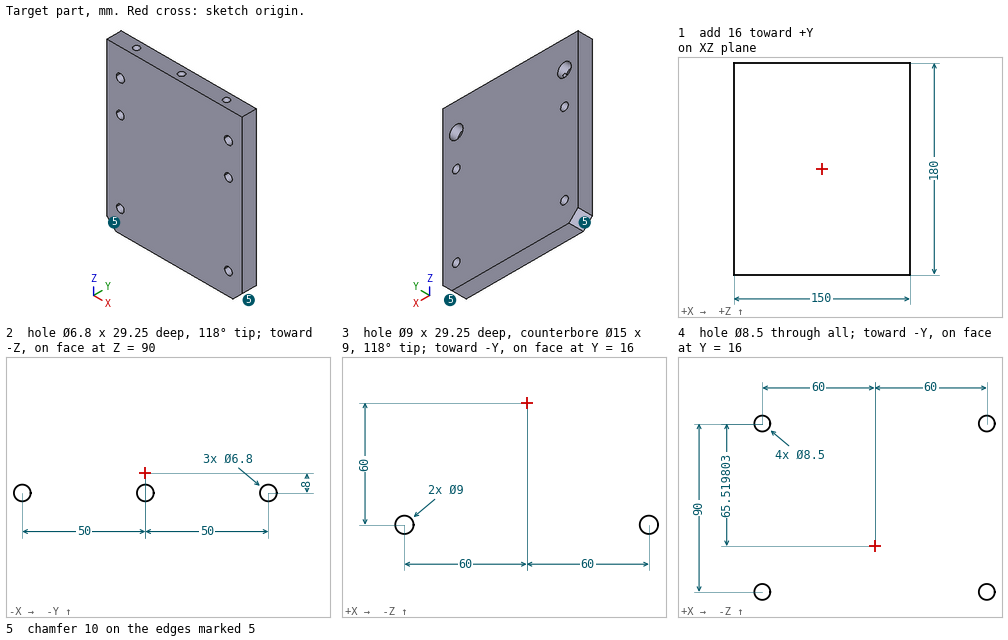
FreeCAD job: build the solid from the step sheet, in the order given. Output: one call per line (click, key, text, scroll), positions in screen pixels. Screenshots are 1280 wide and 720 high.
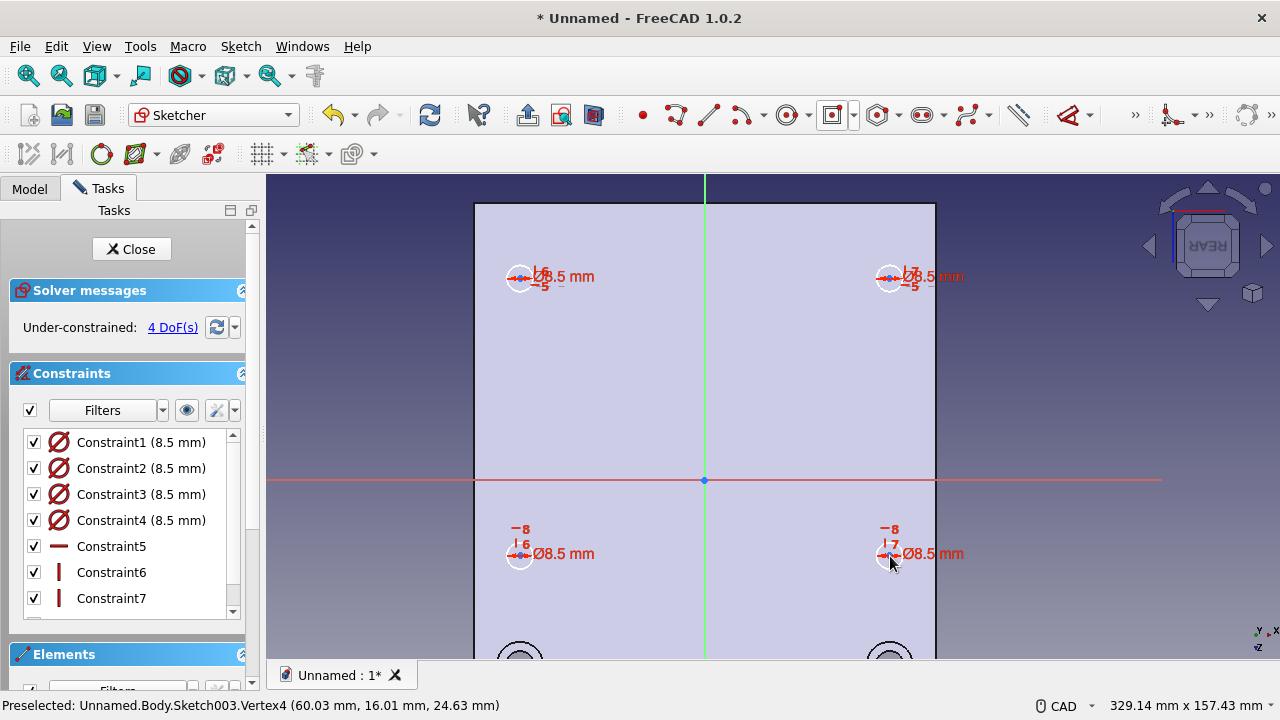
click(1068, 116)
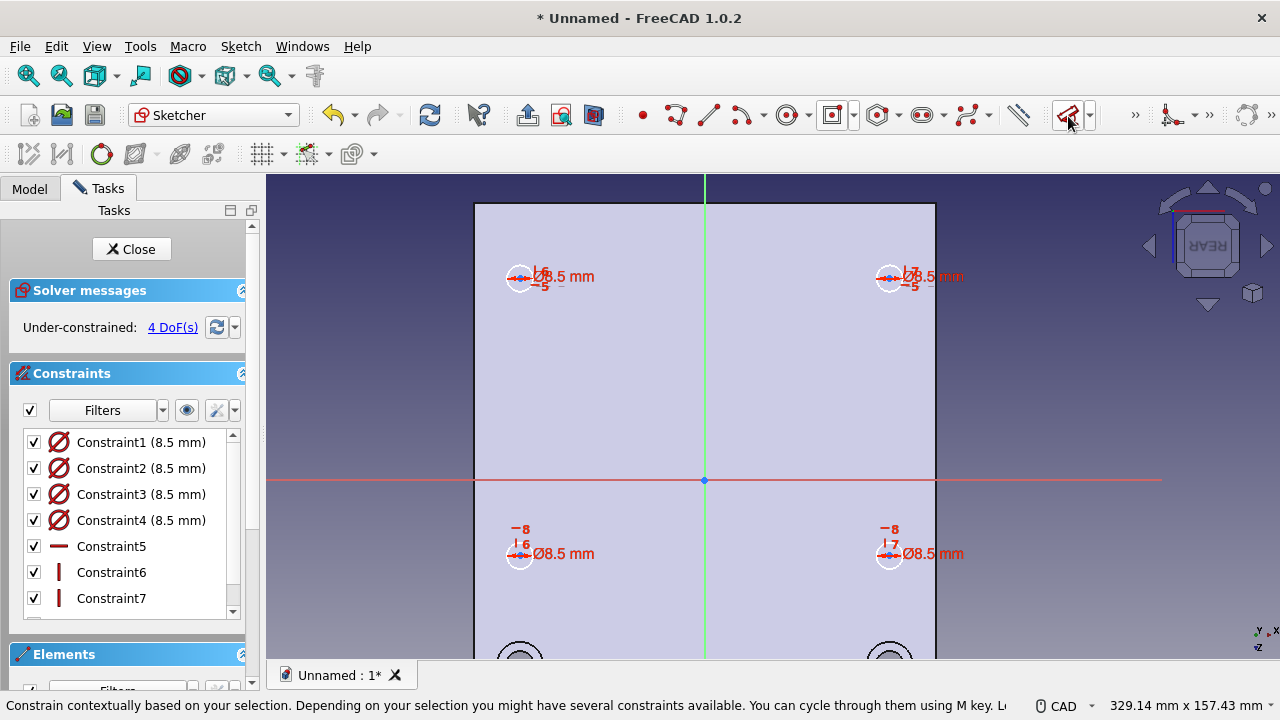
click(520, 279)
click(612, 245)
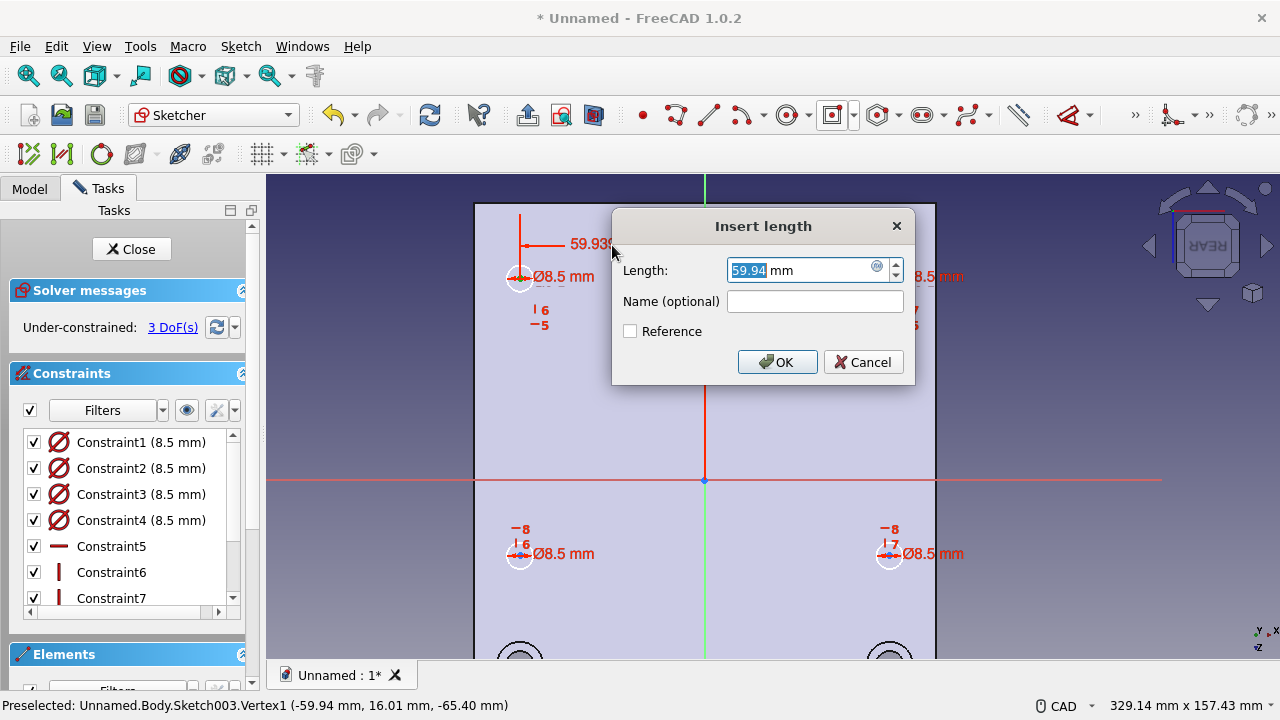
text(60)
key(Return)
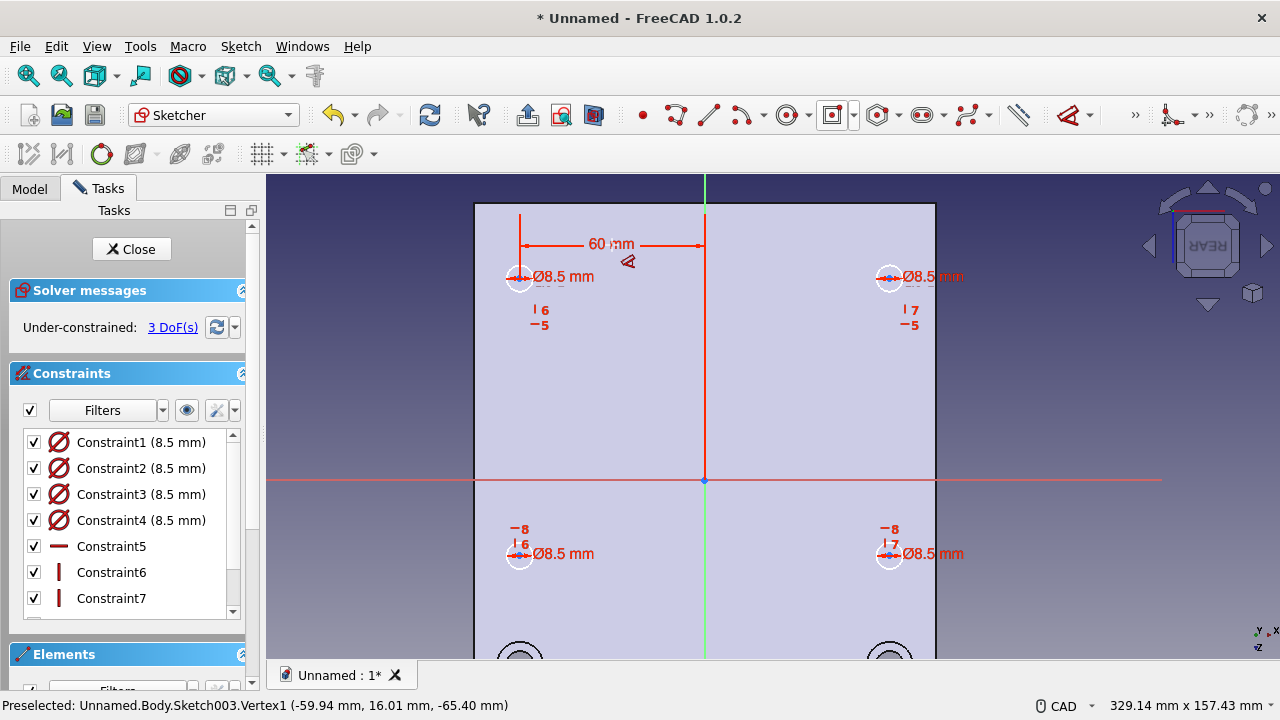
click(890, 279)
click(797, 245)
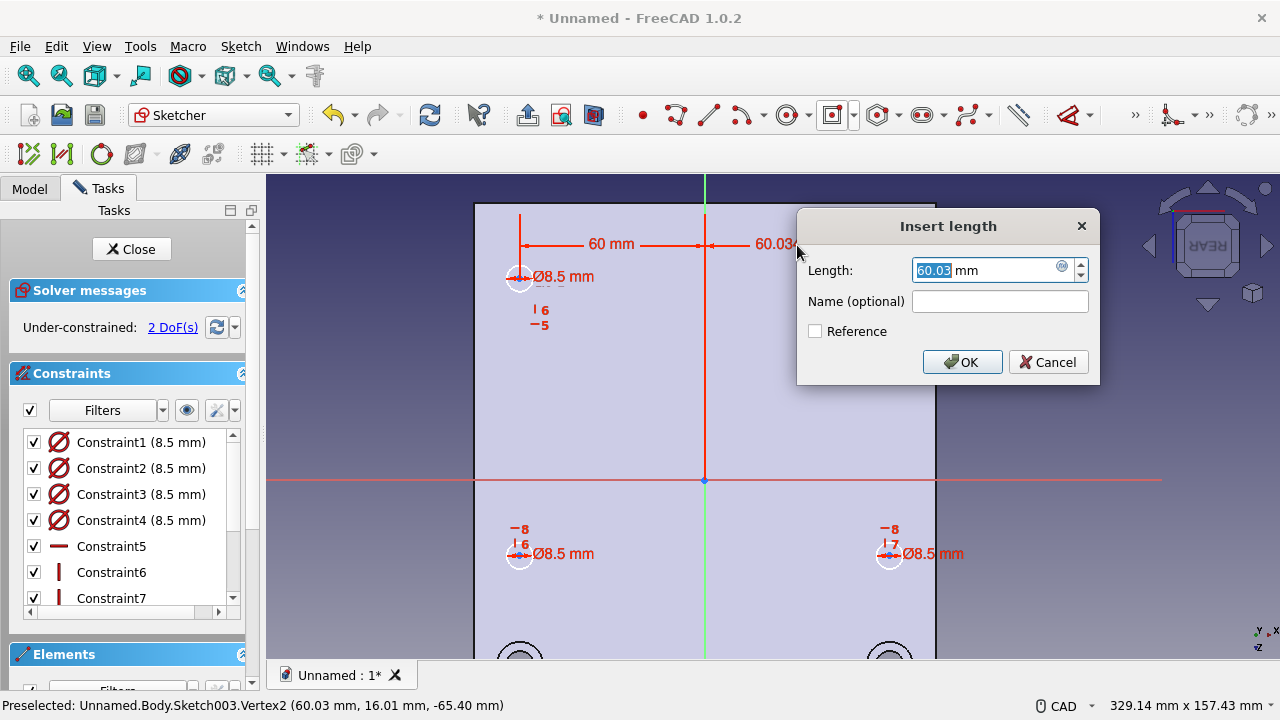
text(60)
key(Return)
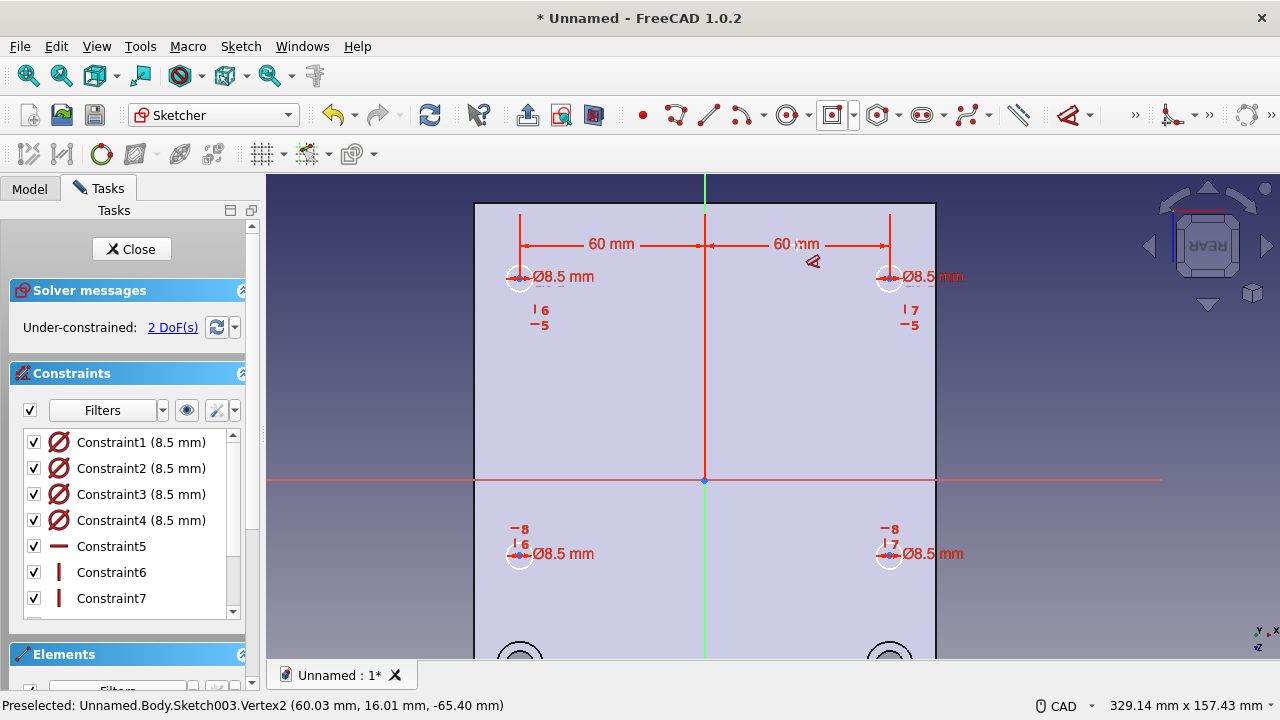
click(520, 279)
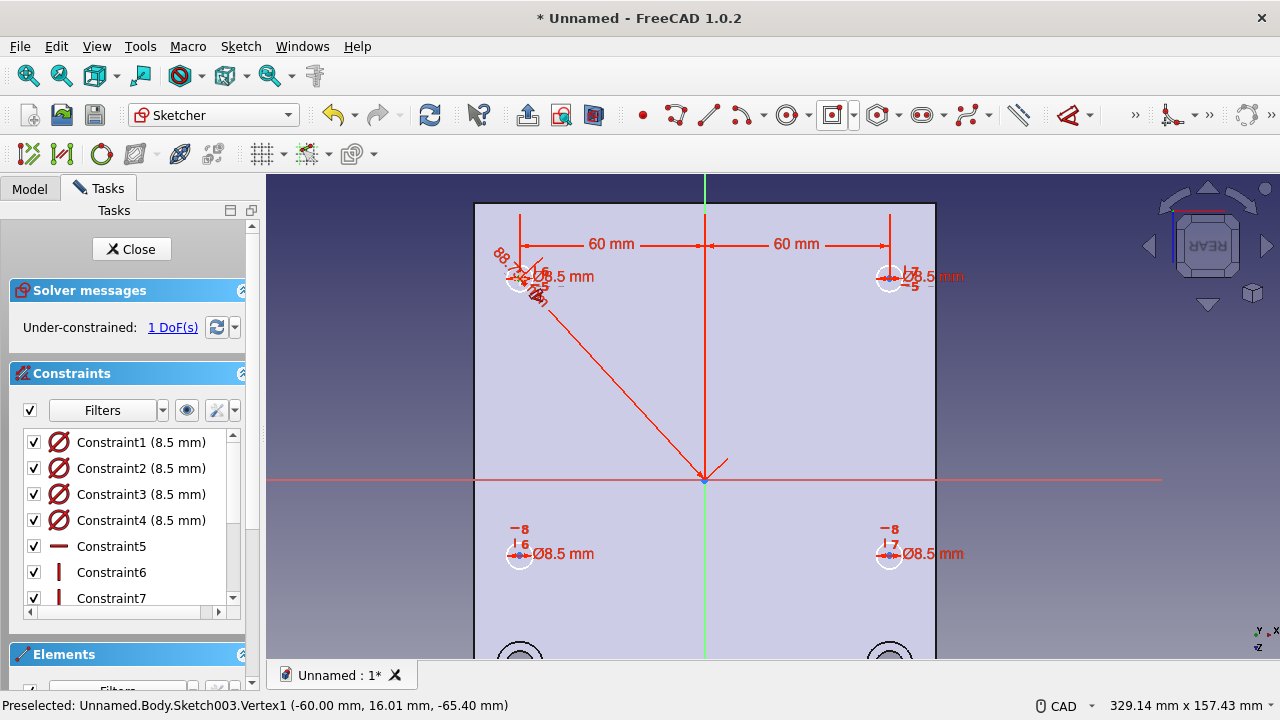
click(520, 556)
click(486, 417)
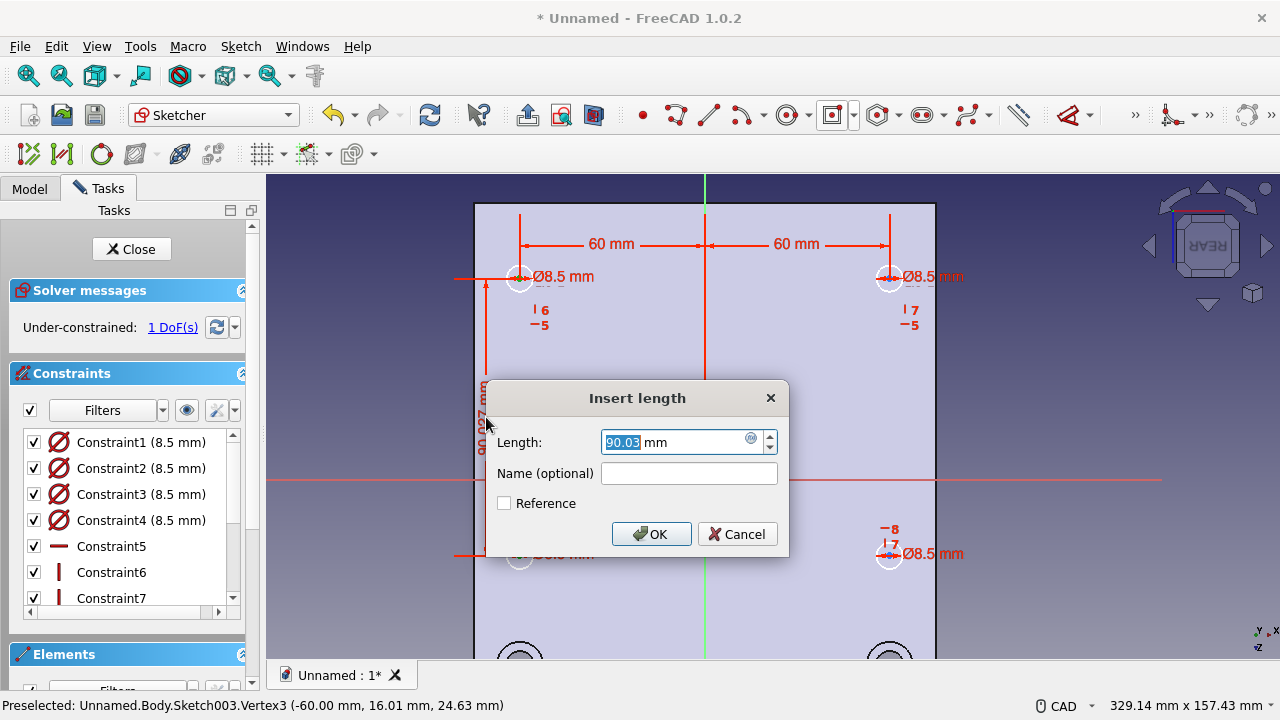
text(90)
key(Return)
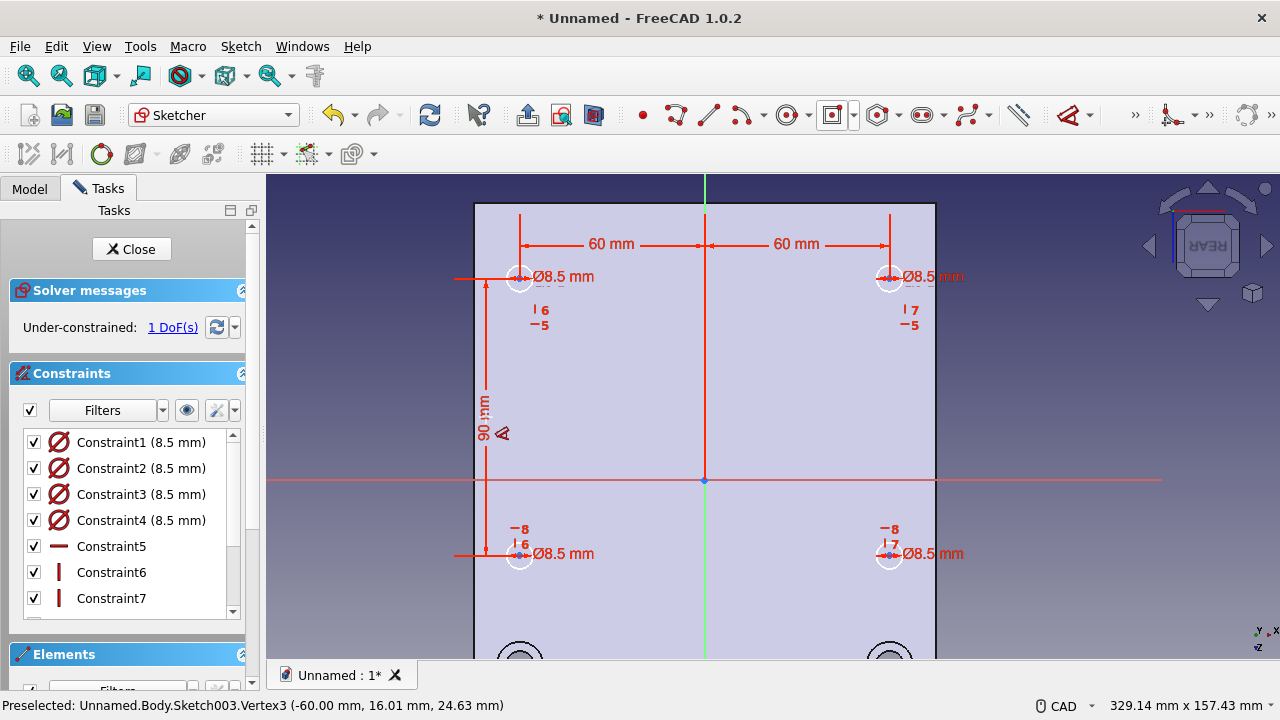
click(520, 279)
click(486, 379)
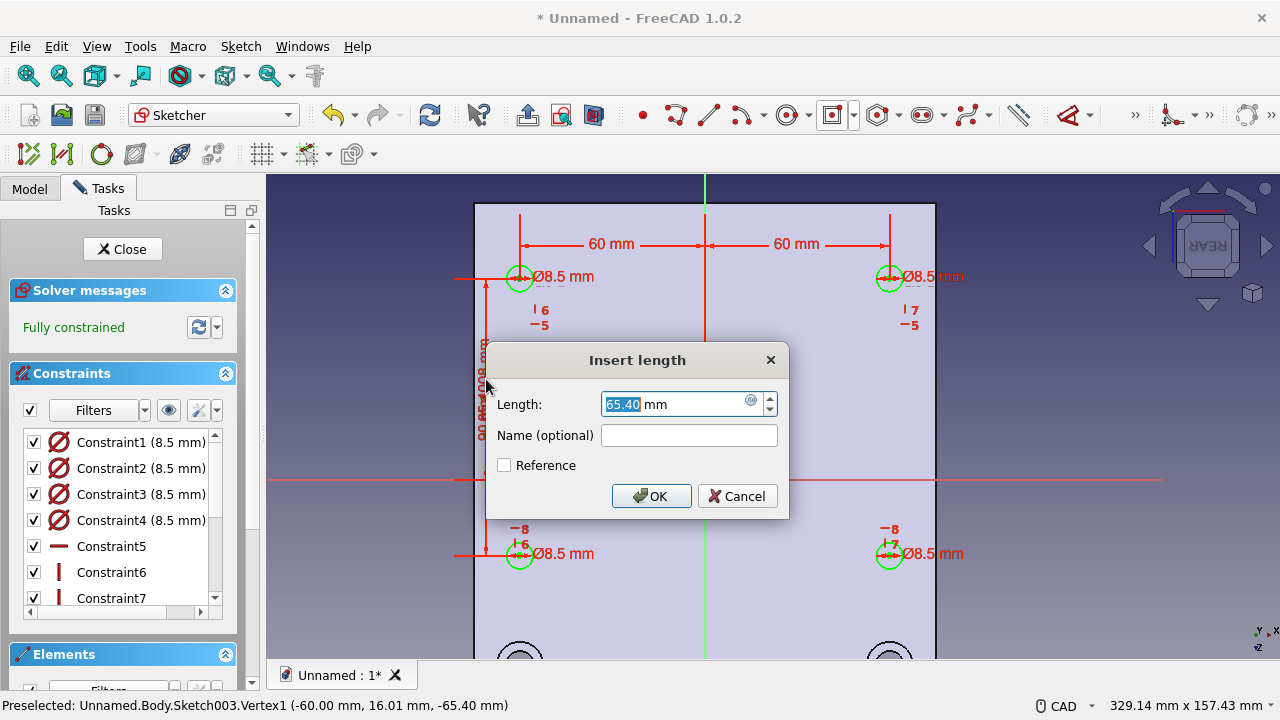
text(65.519803)
key(Return)
key(Escape)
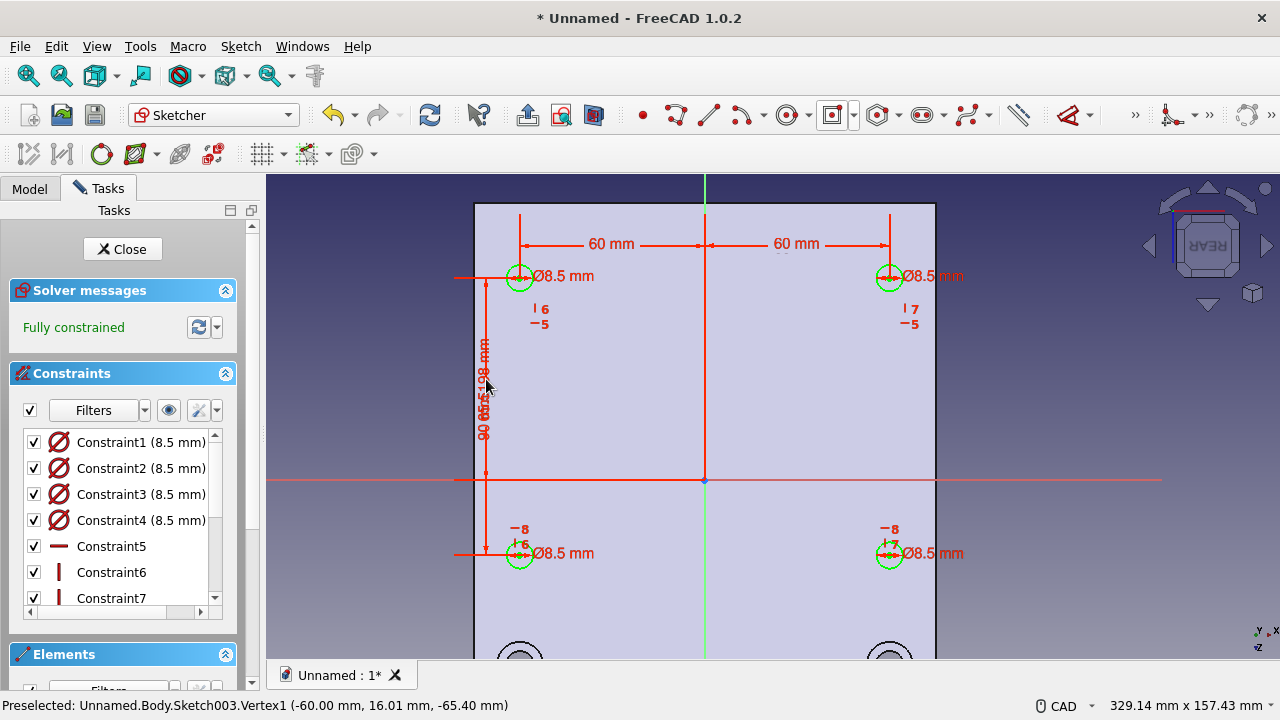
click(123, 249)